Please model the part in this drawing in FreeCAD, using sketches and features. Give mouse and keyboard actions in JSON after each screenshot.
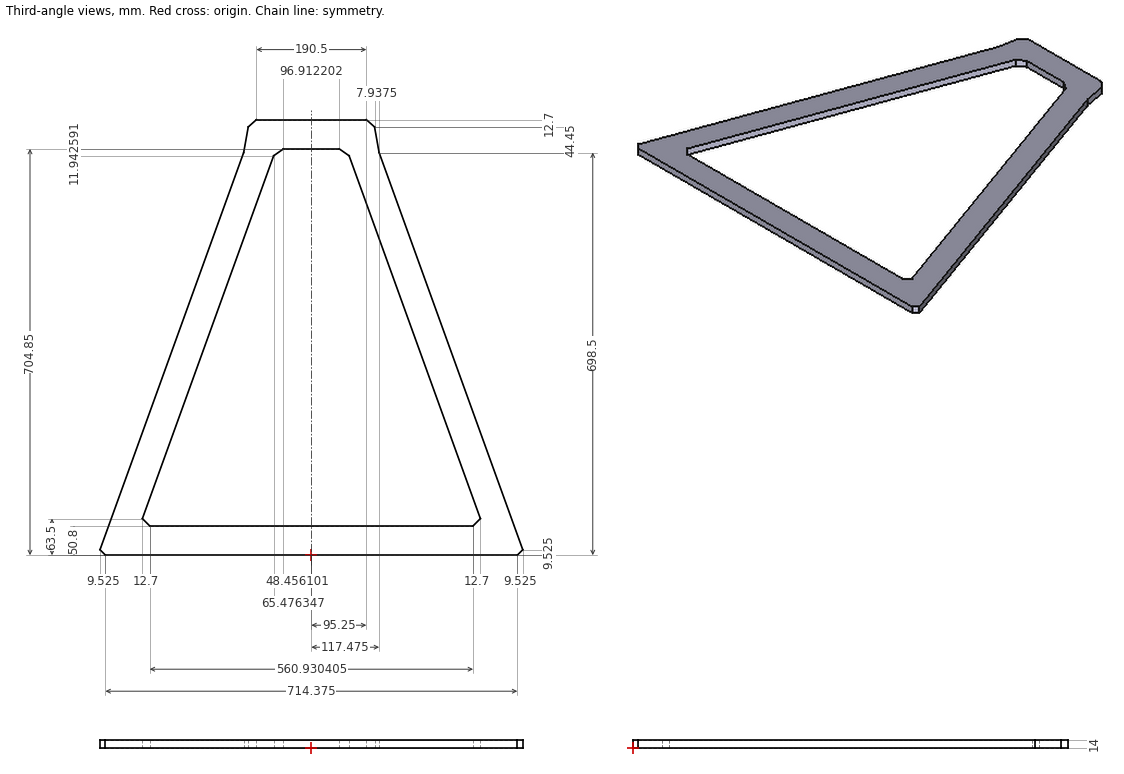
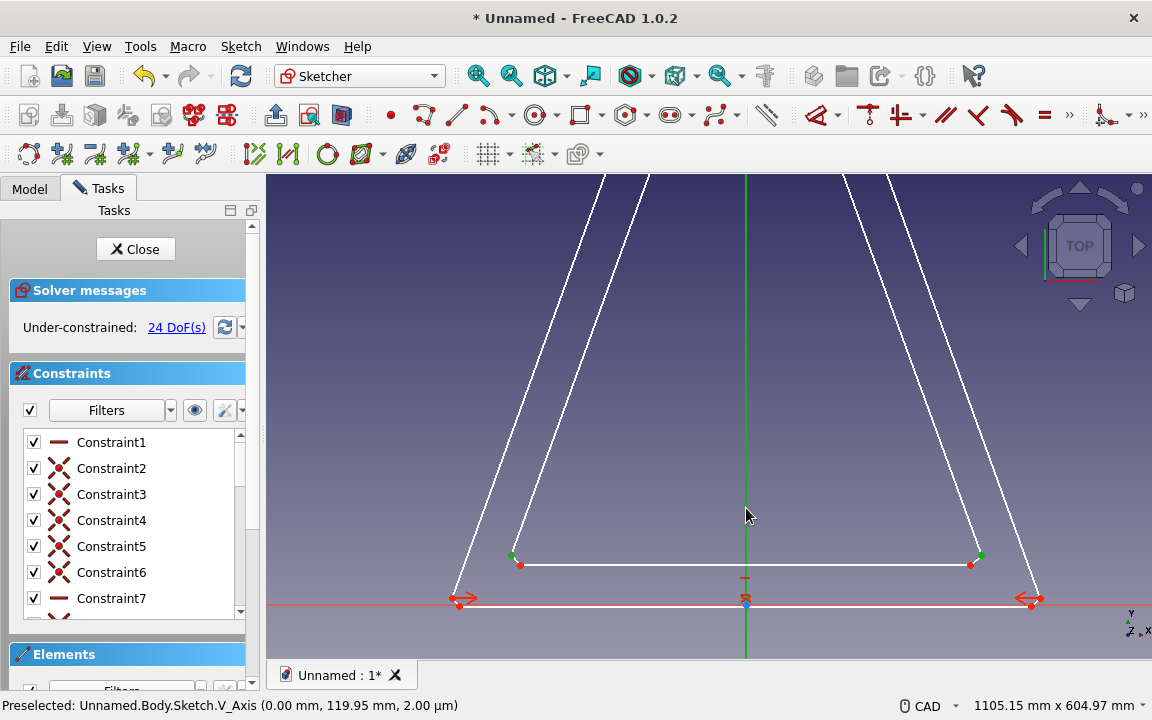
{"action": "key", "text": "s"}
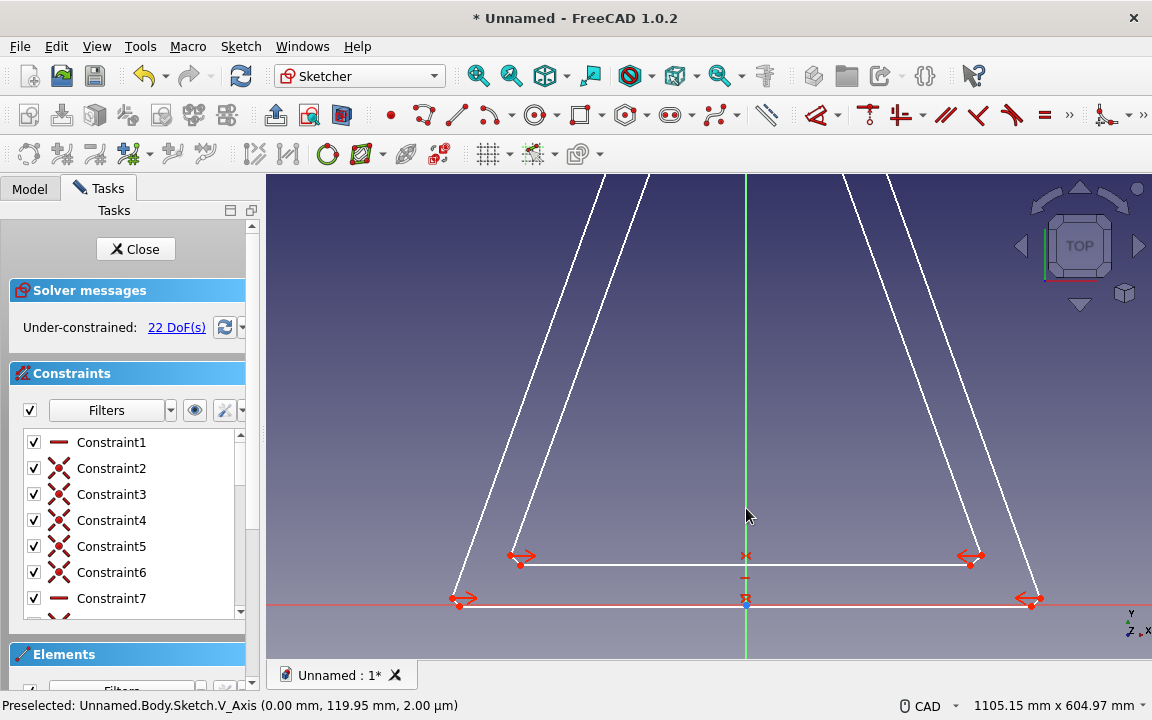
{"action": "left_click", "coordinate": [460, 607]}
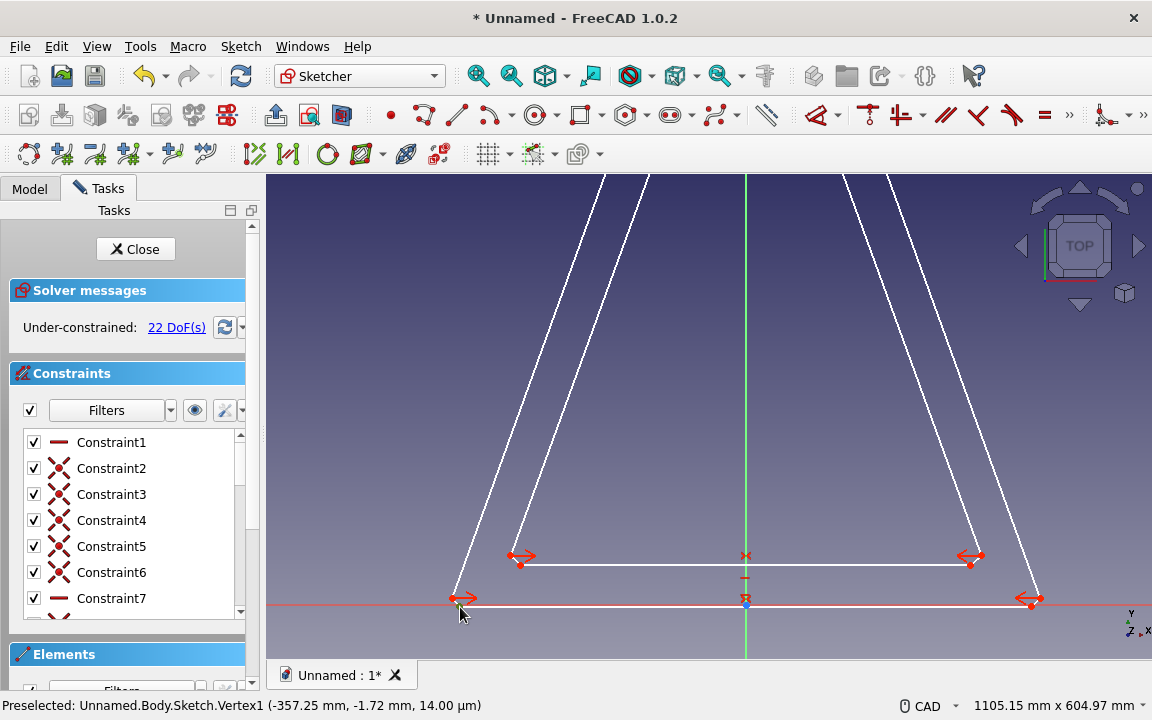
{"action": "left_click", "coordinate": [344, 605]}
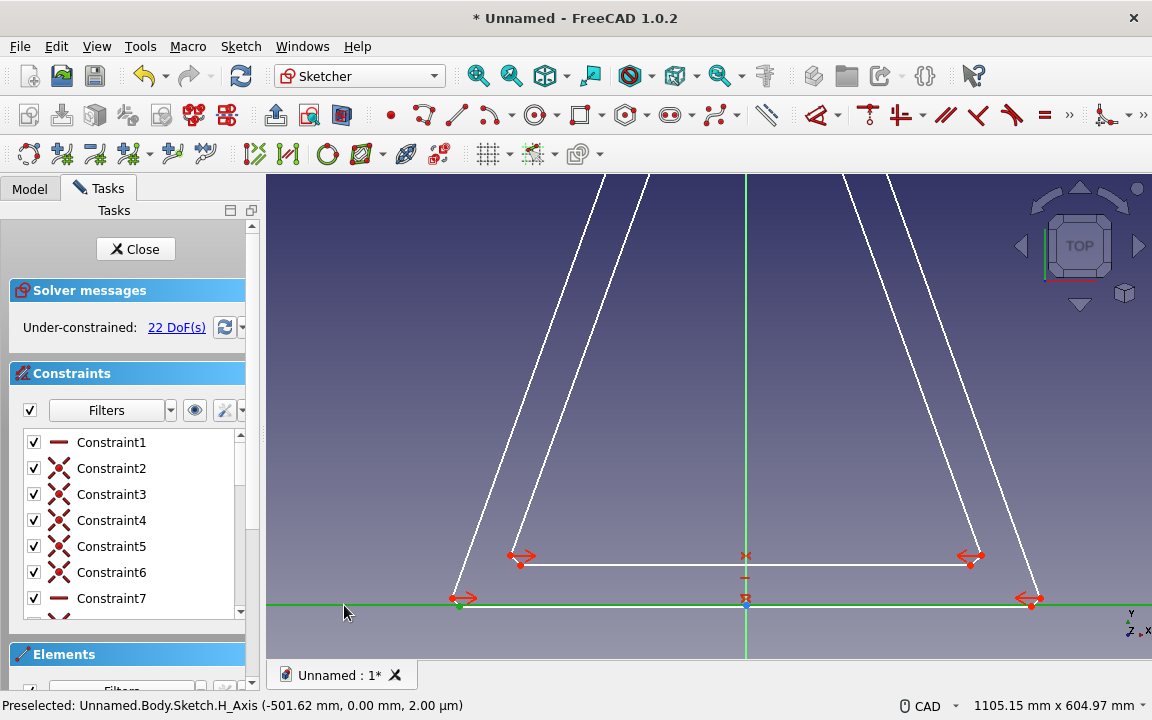
{"action": "left_click", "coordinate": [868, 116]}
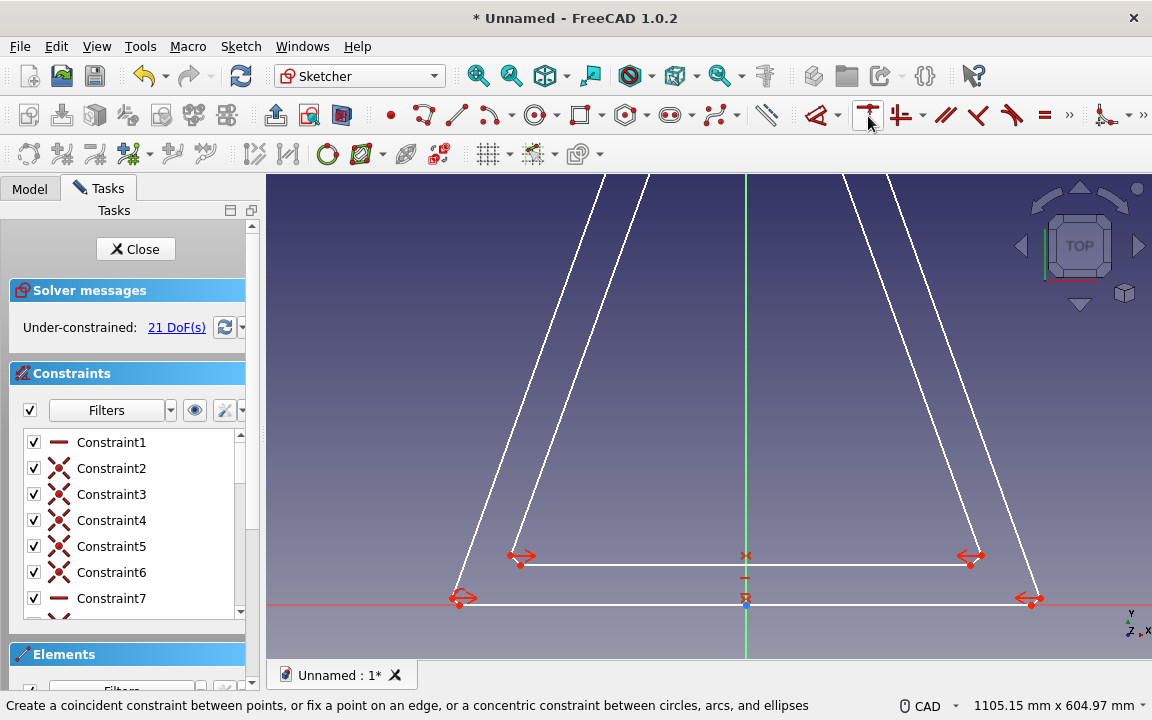
{"action": "key", "text": "d"}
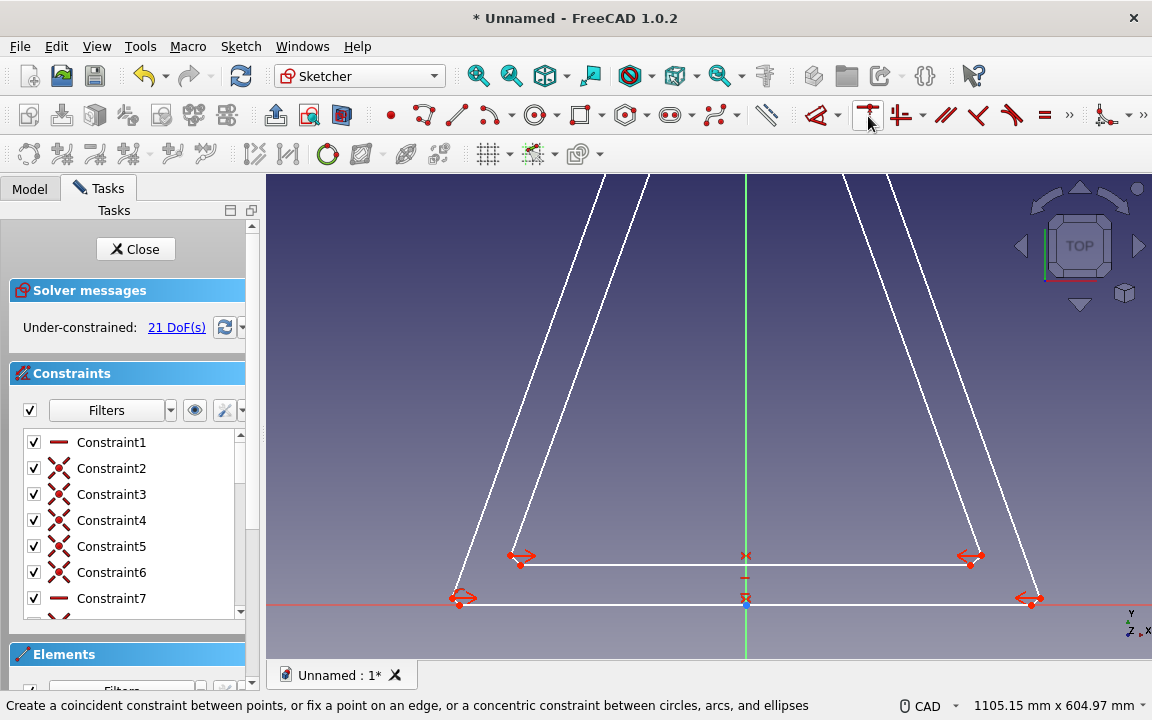
{"action": "scroll", "coordinate": [512, 555], "scroll_direction": "down", "scroll_amount": 3}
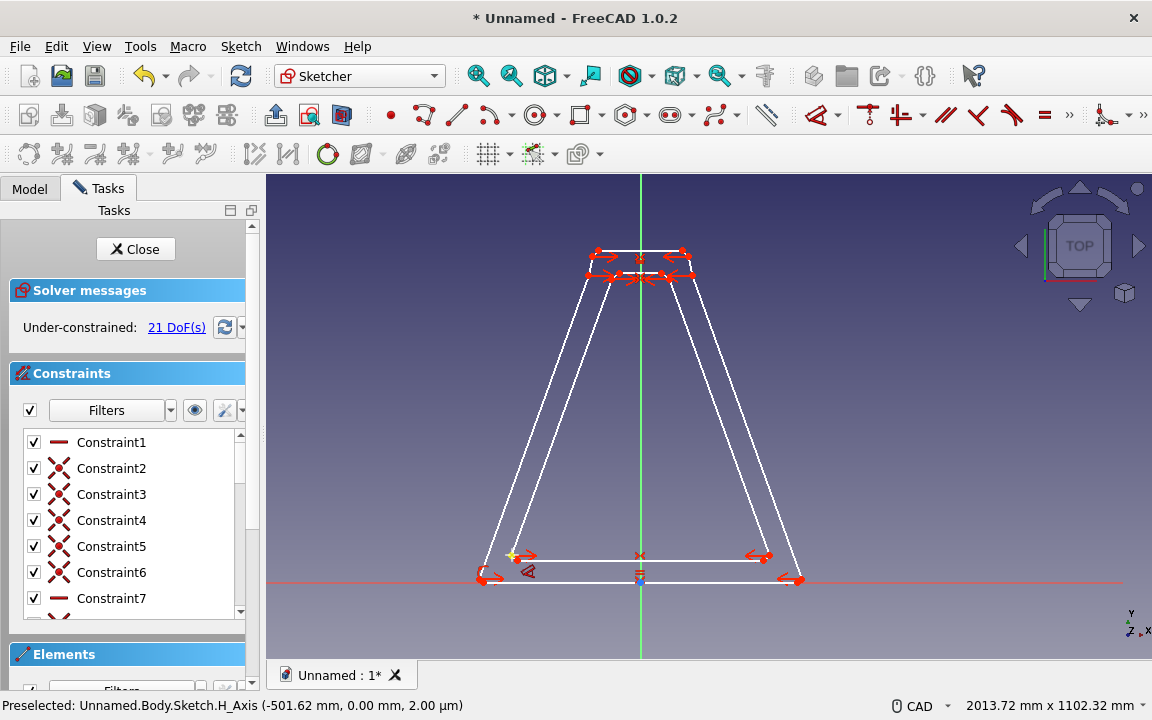
{"action": "left_click", "coordinate": [658, 251]}
{"action": "left_click", "coordinate": [621, 217]}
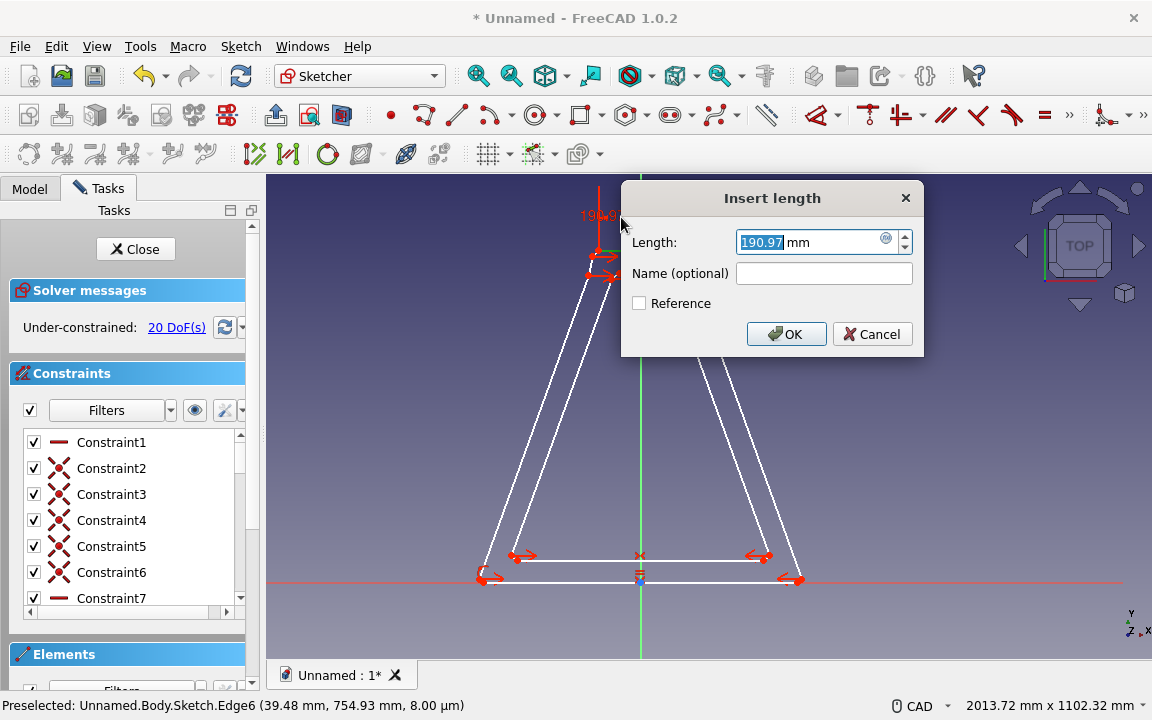
{"action": "type", "text": "190.5"}
{"action": "key", "text": "Return"}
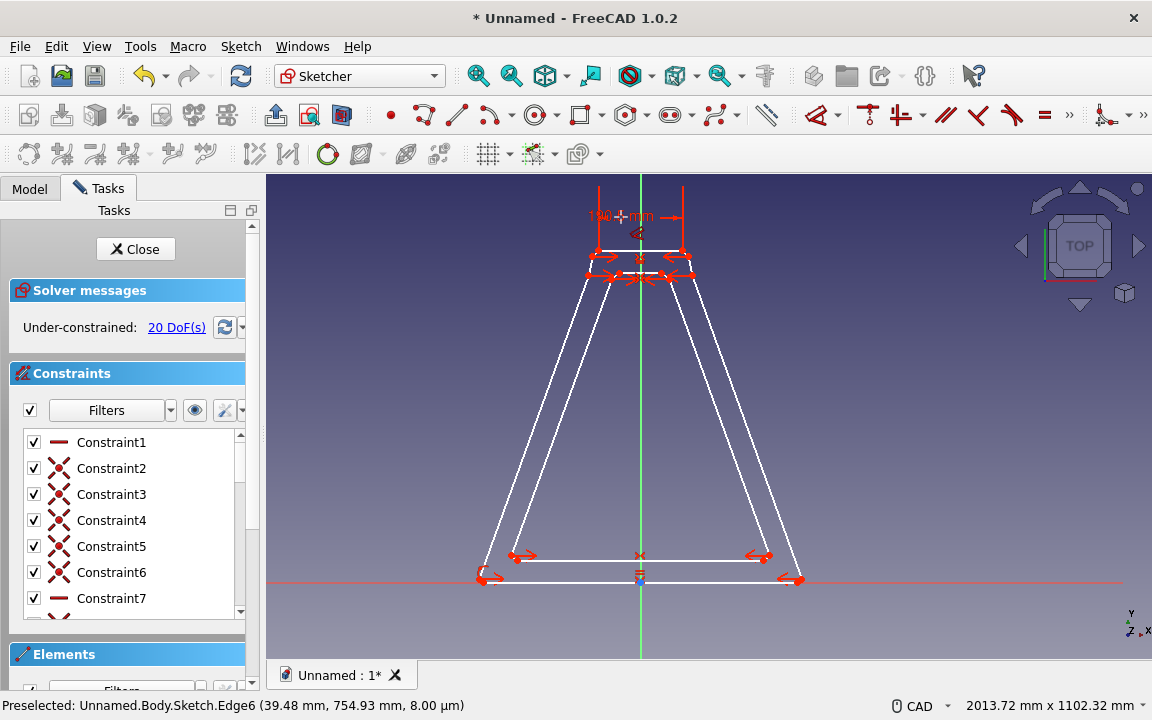
{"action": "scroll", "coordinate": [517, 561], "scroll_direction": "up", "scroll_amount": 3}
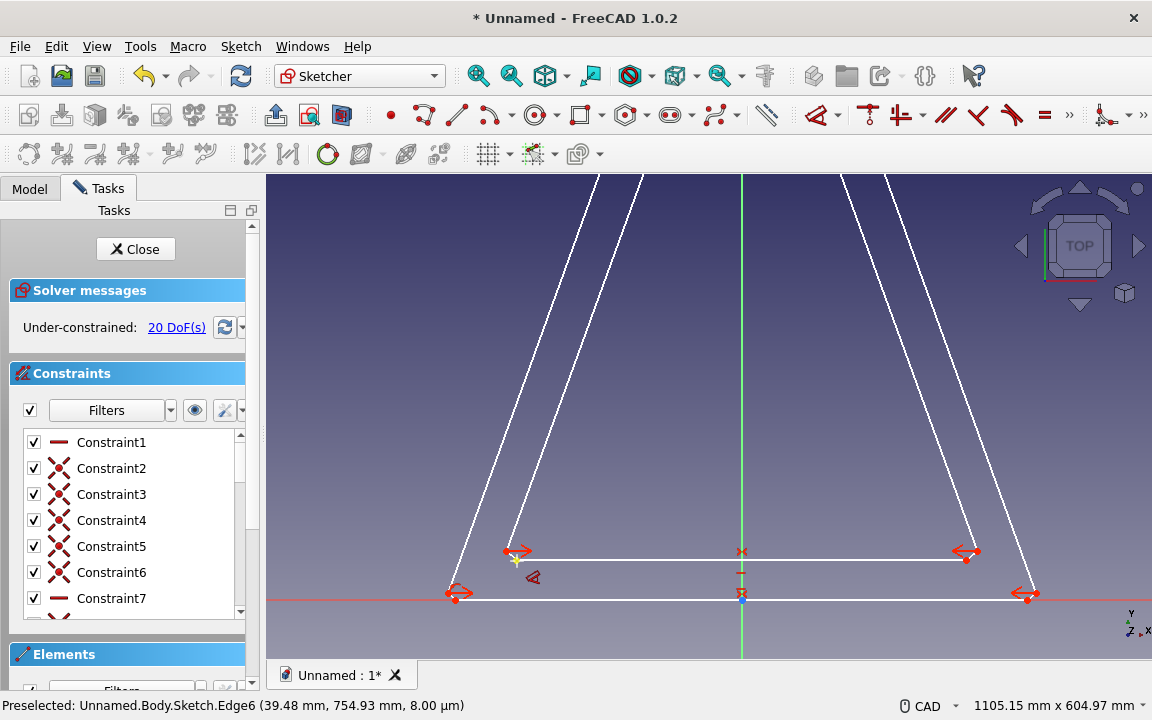
{"action": "left_click", "coordinate": [517, 560]}
{"action": "left_click", "coordinate": [483, 580]}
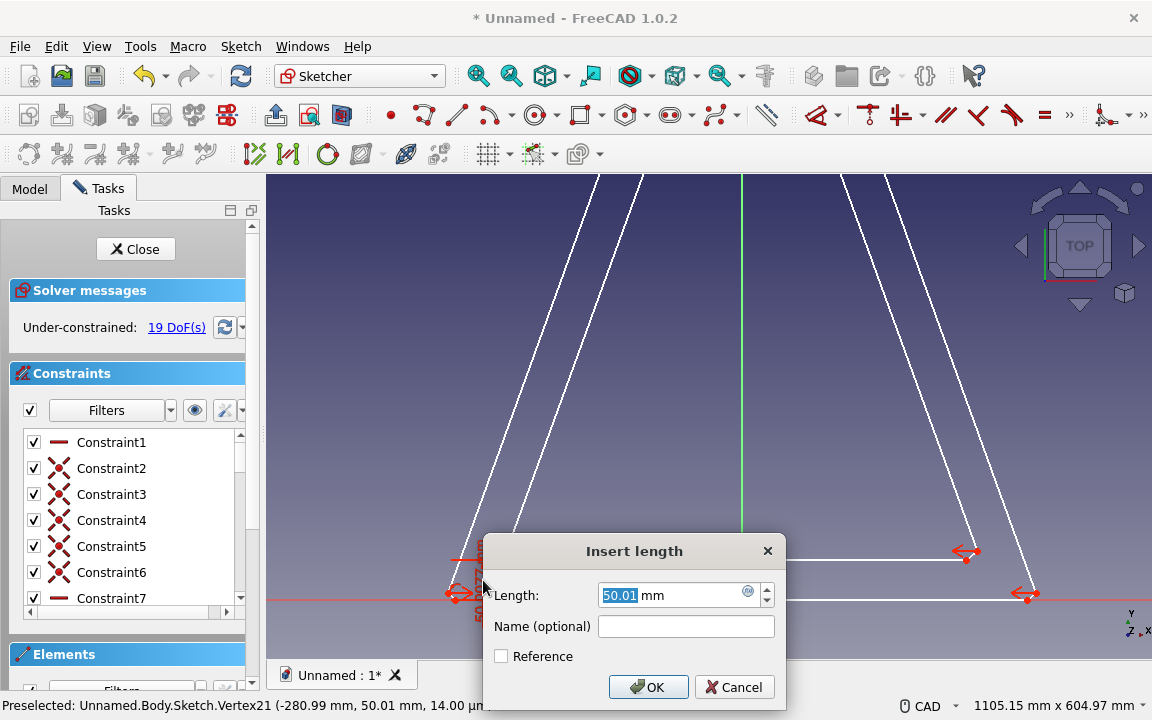
{"action": "type", "text": "50.8"}
{"action": "key", "text": "Return"}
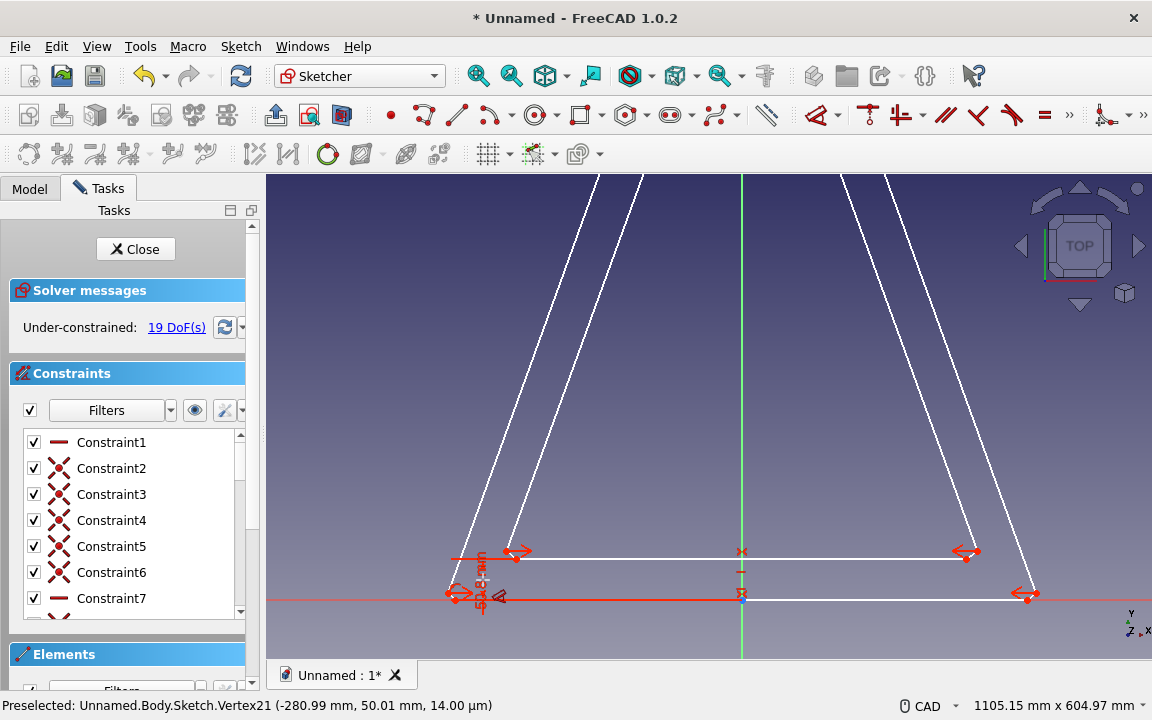
{"action": "left_click", "coordinate": [507, 551]}
{"action": "left_click", "coordinate": [776, 576]}